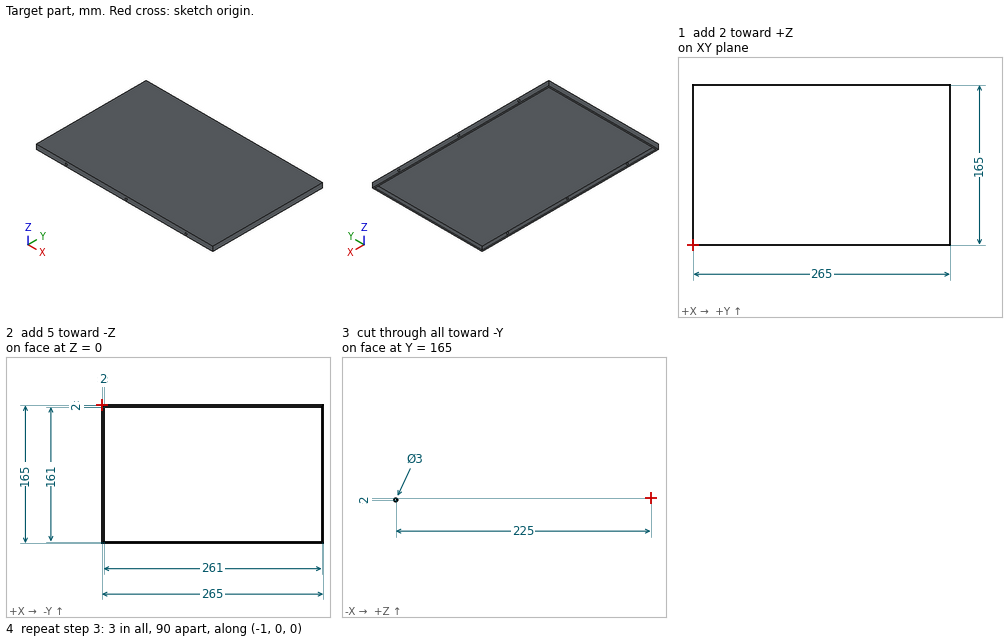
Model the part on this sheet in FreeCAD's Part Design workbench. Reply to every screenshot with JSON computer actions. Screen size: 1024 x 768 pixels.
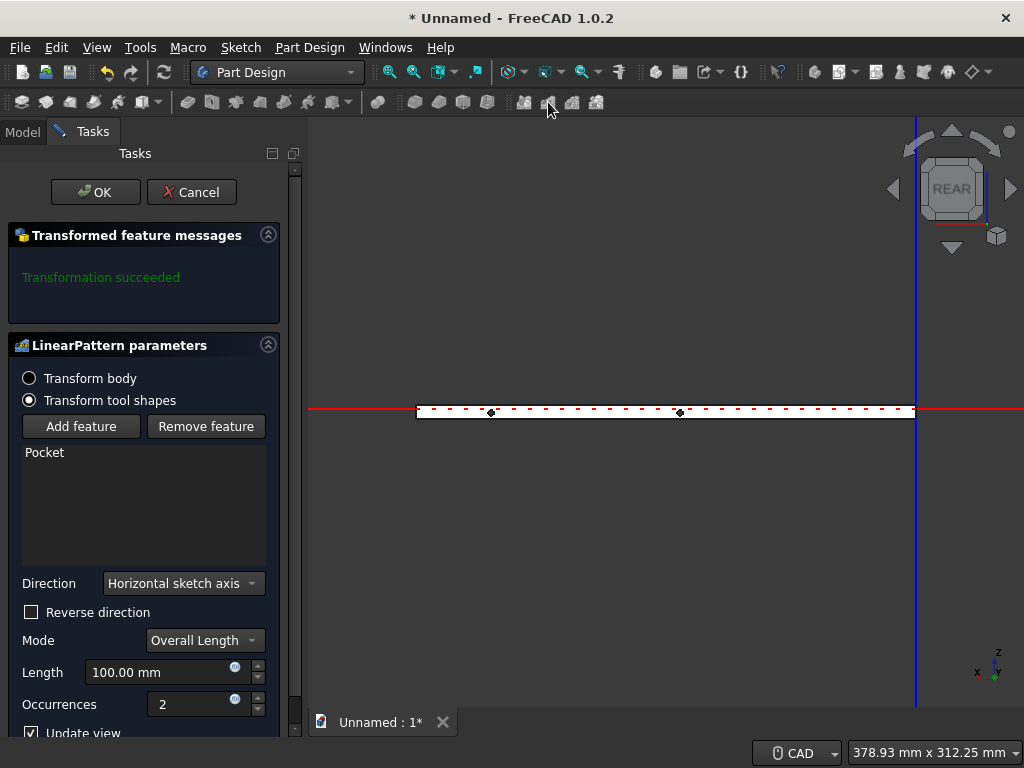
{"action": "left_click", "coordinate": [184, 584]}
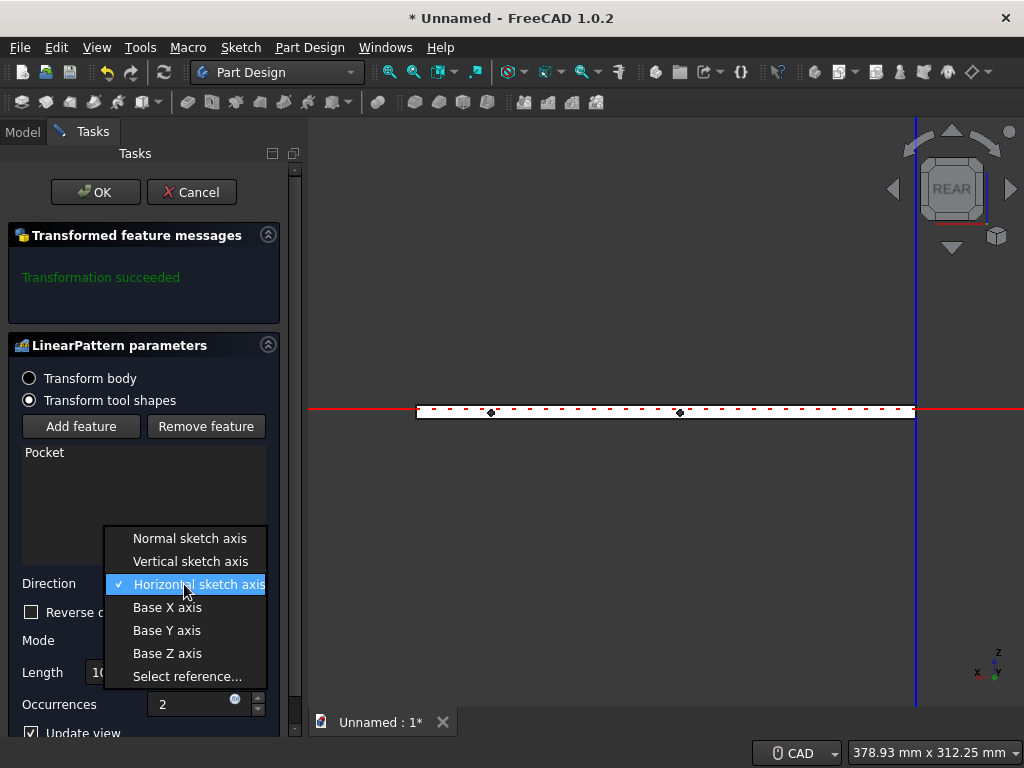
{"action": "left_click", "coordinate": [184, 608]}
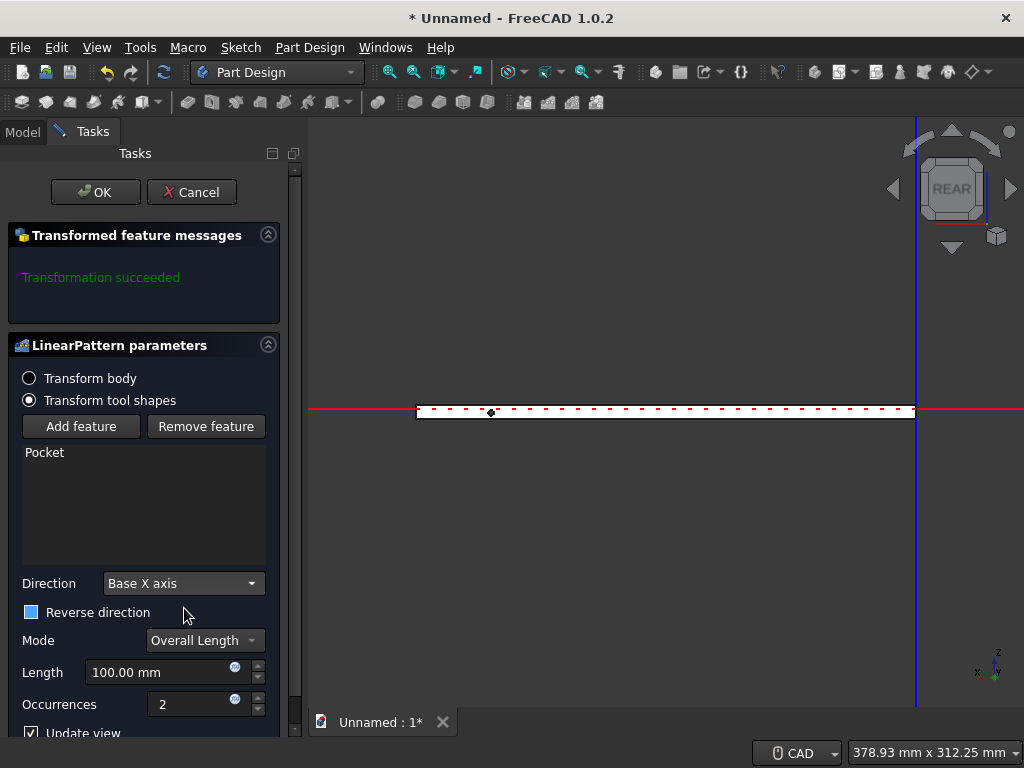
{"action": "left_click", "coordinate": [206, 640]}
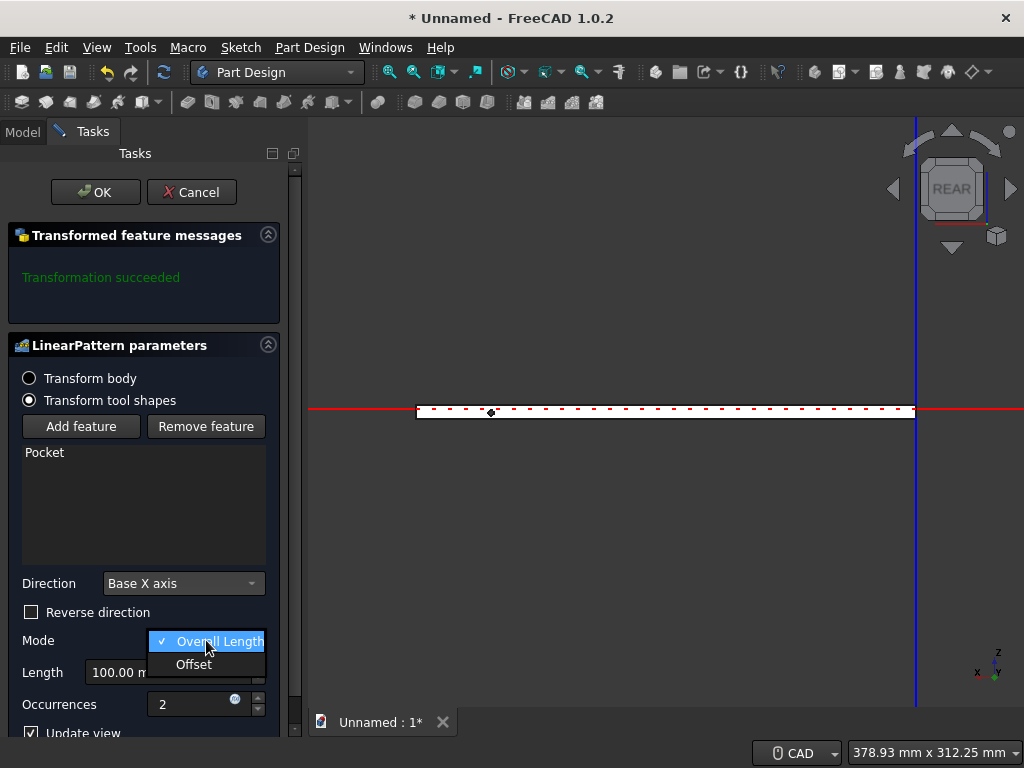
{"action": "left_click", "coordinate": [206, 664]}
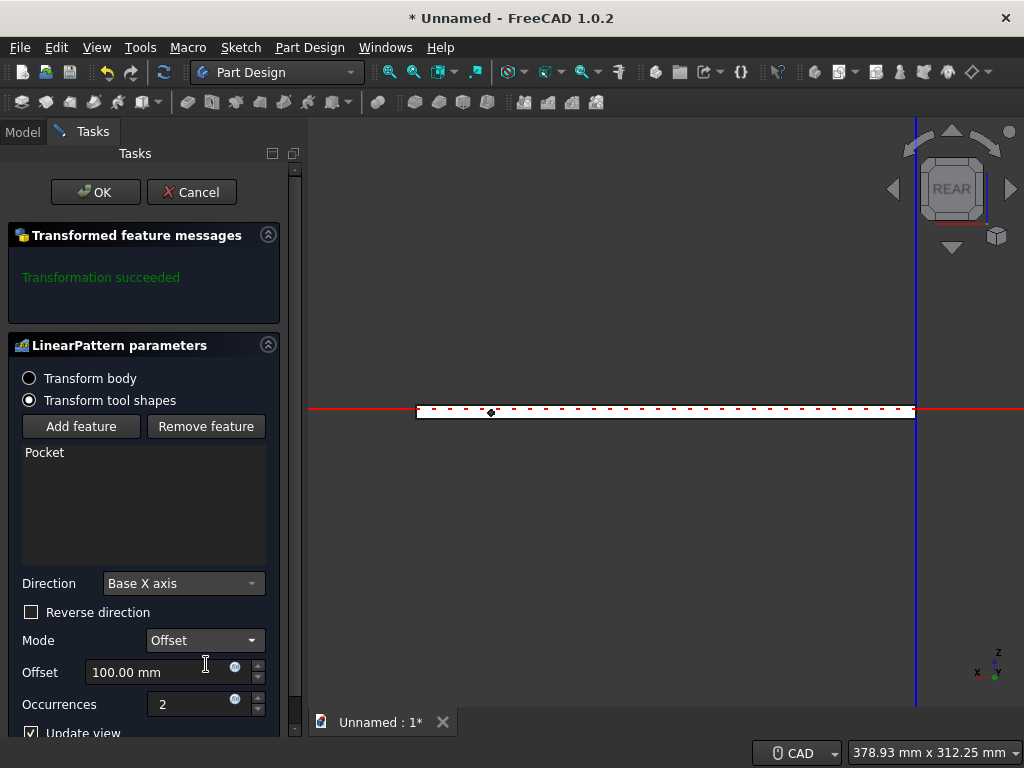
{"action": "triple_click", "coordinate": [168, 672]}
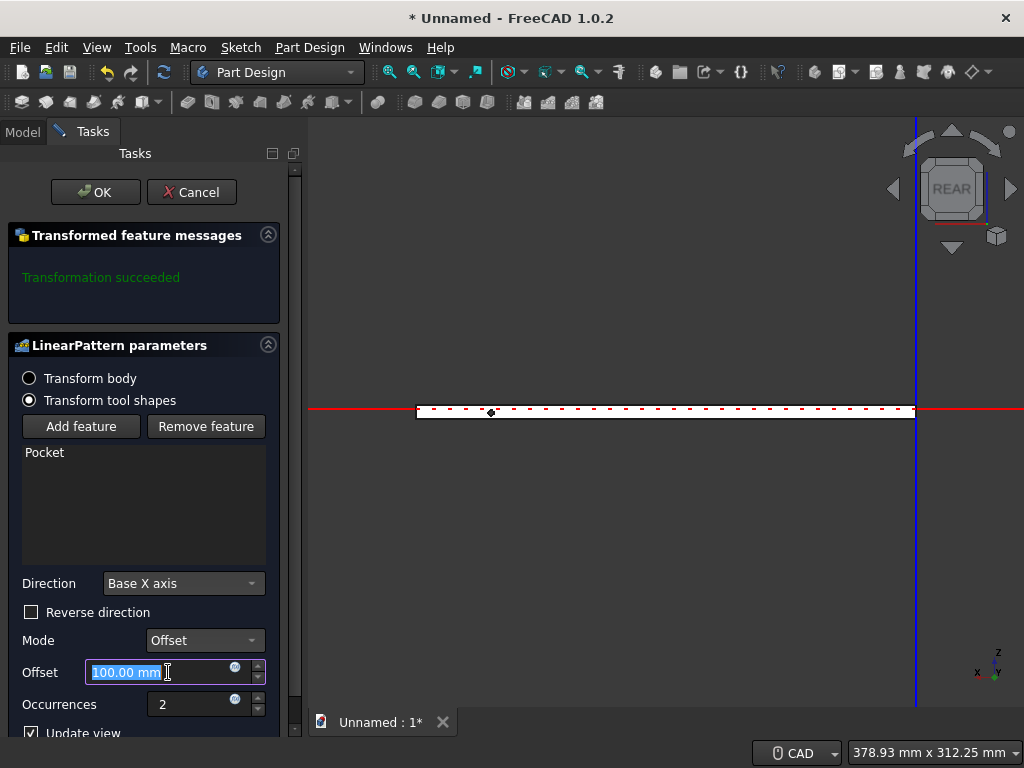
{"action": "type", "text": "90"}
{"action": "key", "text": "Tab"}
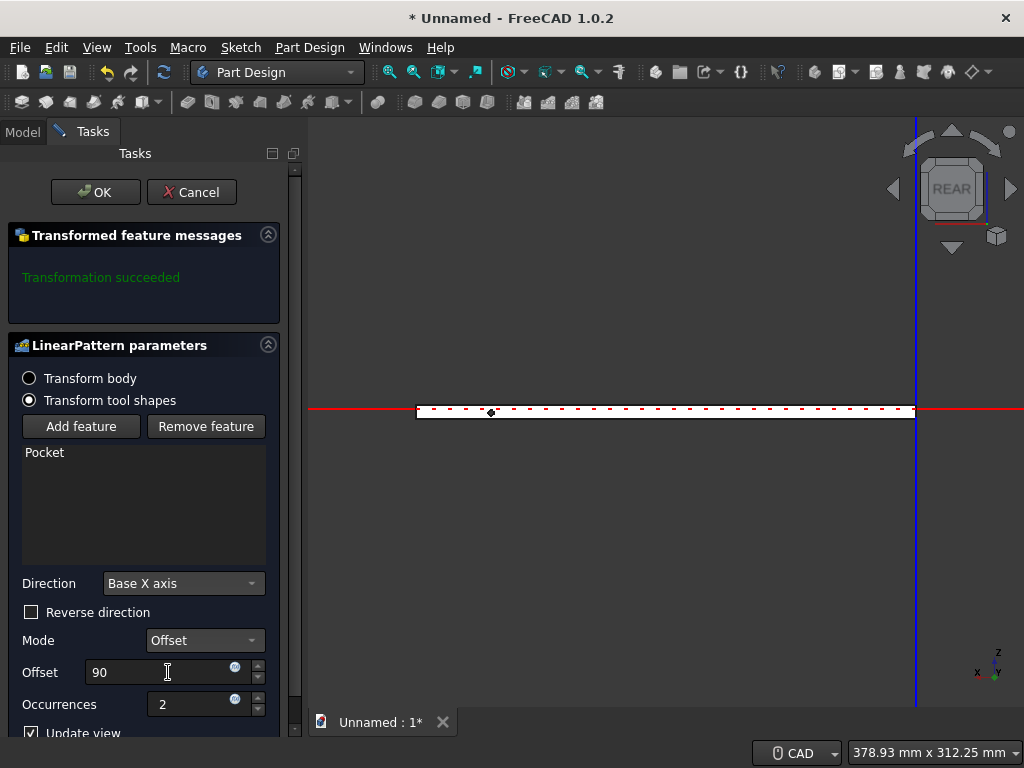
{"action": "triple_click", "coordinate": [198, 704]}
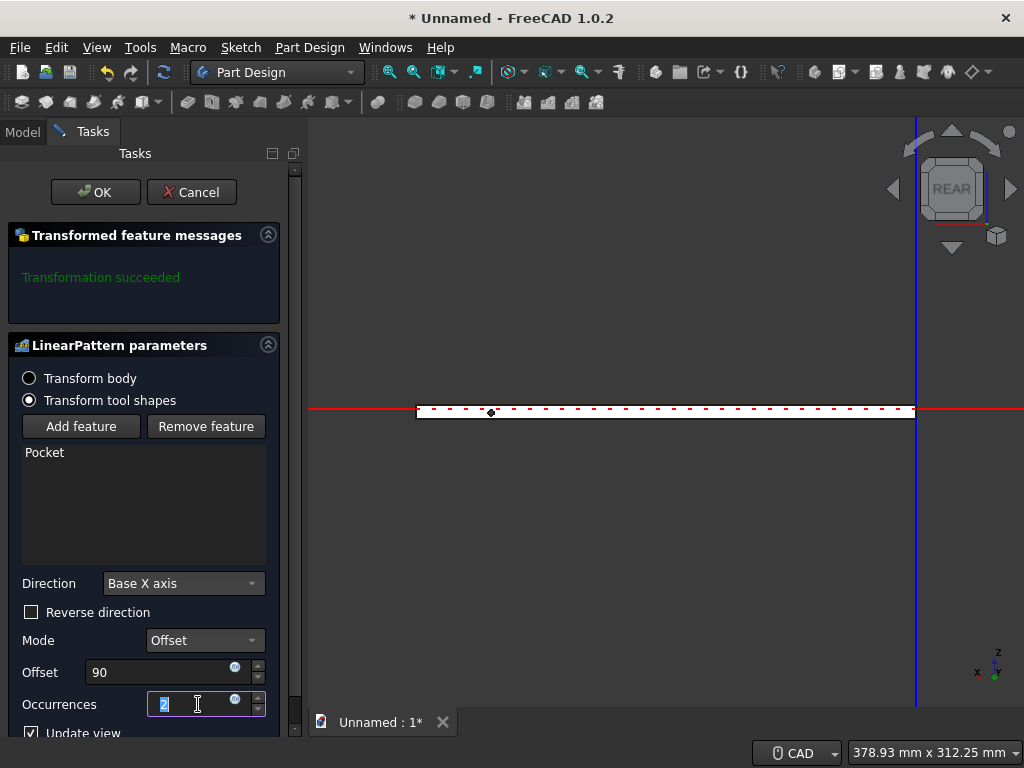
{"action": "type", "text": "3"}
{"action": "key", "text": "Tab"}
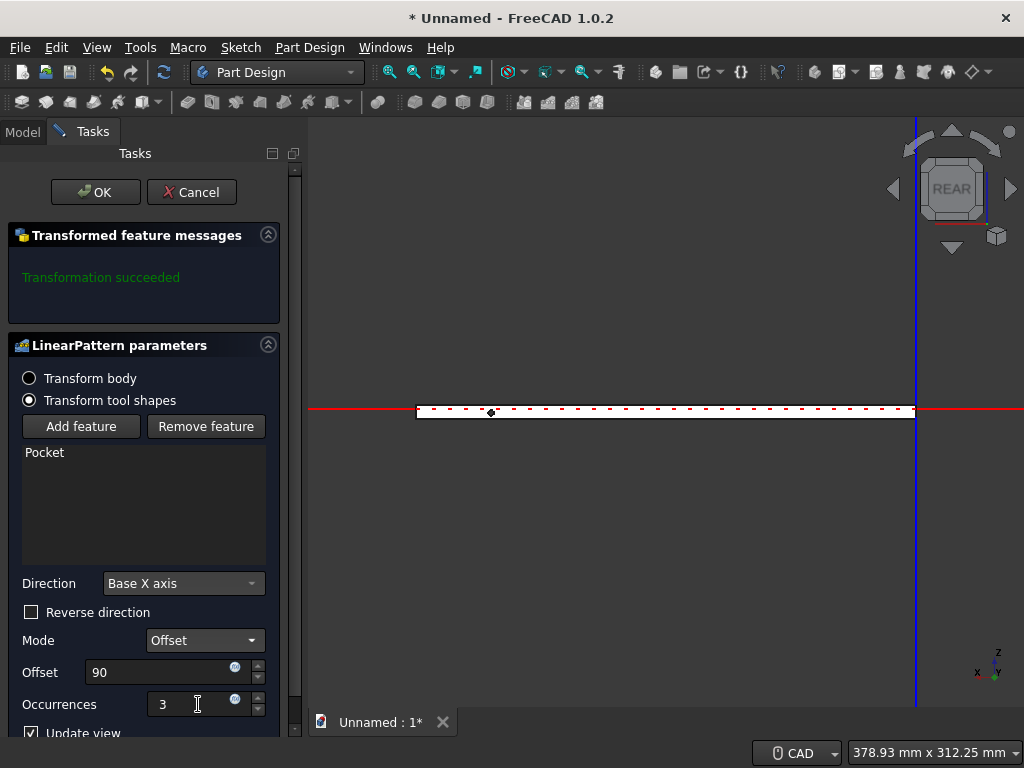
{"action": "left_click", "coordinate": [30, 612]}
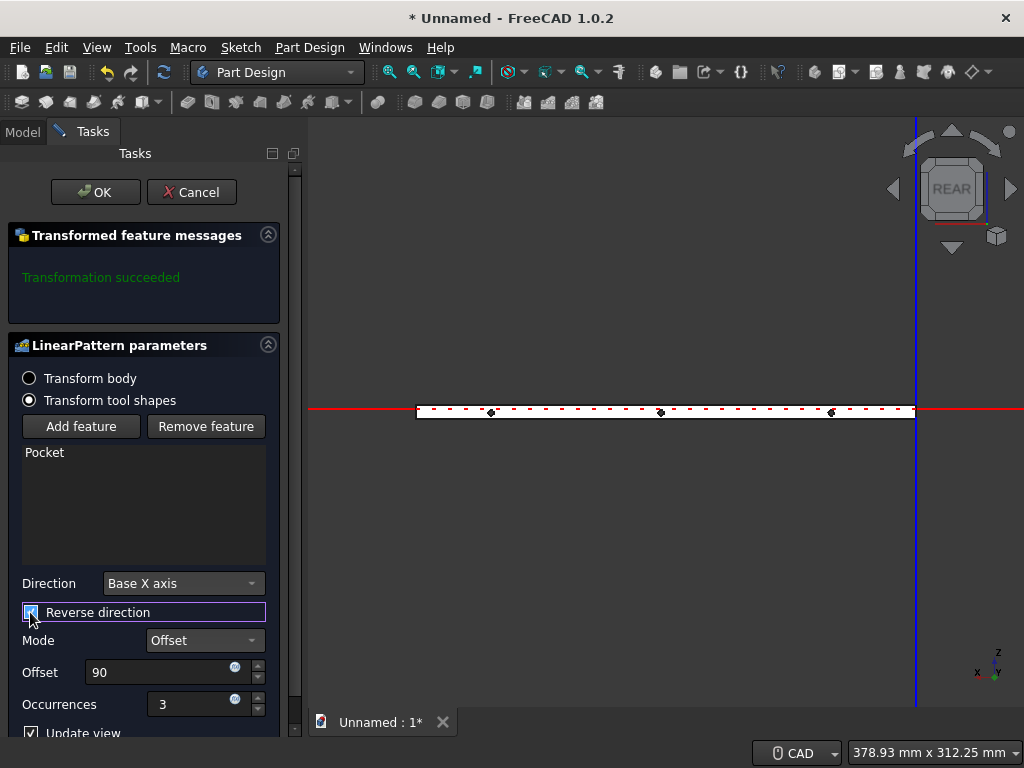
{"action": "left_click", "coordinate": [96, 192]}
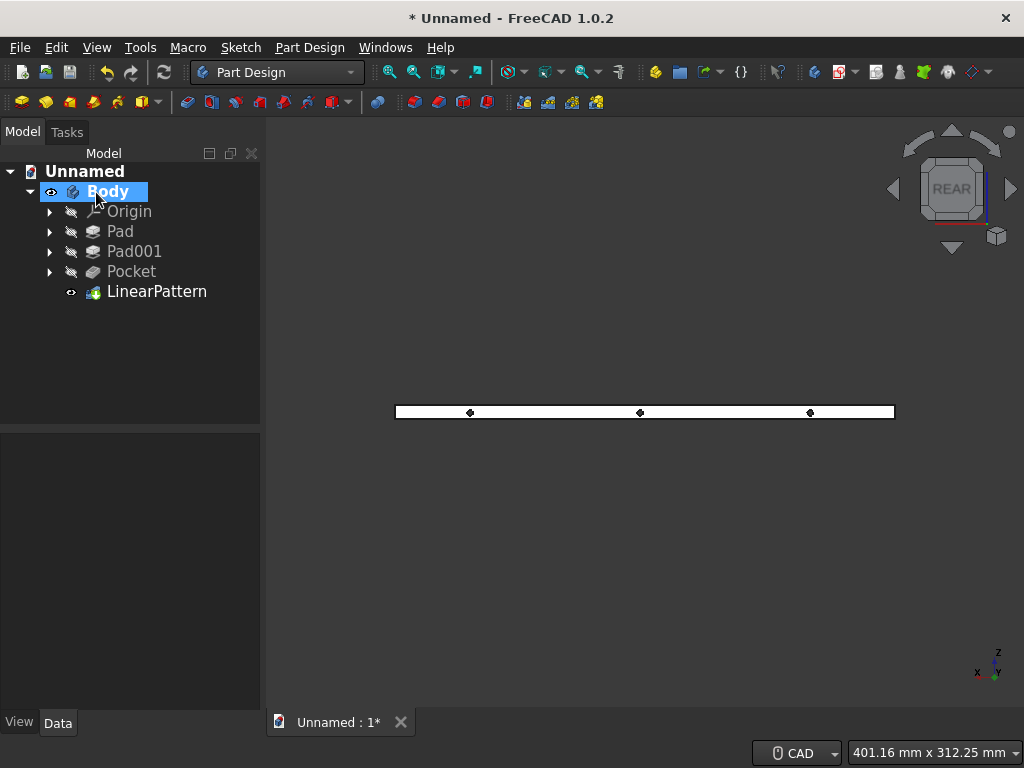
{"action": "key", "text": "0"}